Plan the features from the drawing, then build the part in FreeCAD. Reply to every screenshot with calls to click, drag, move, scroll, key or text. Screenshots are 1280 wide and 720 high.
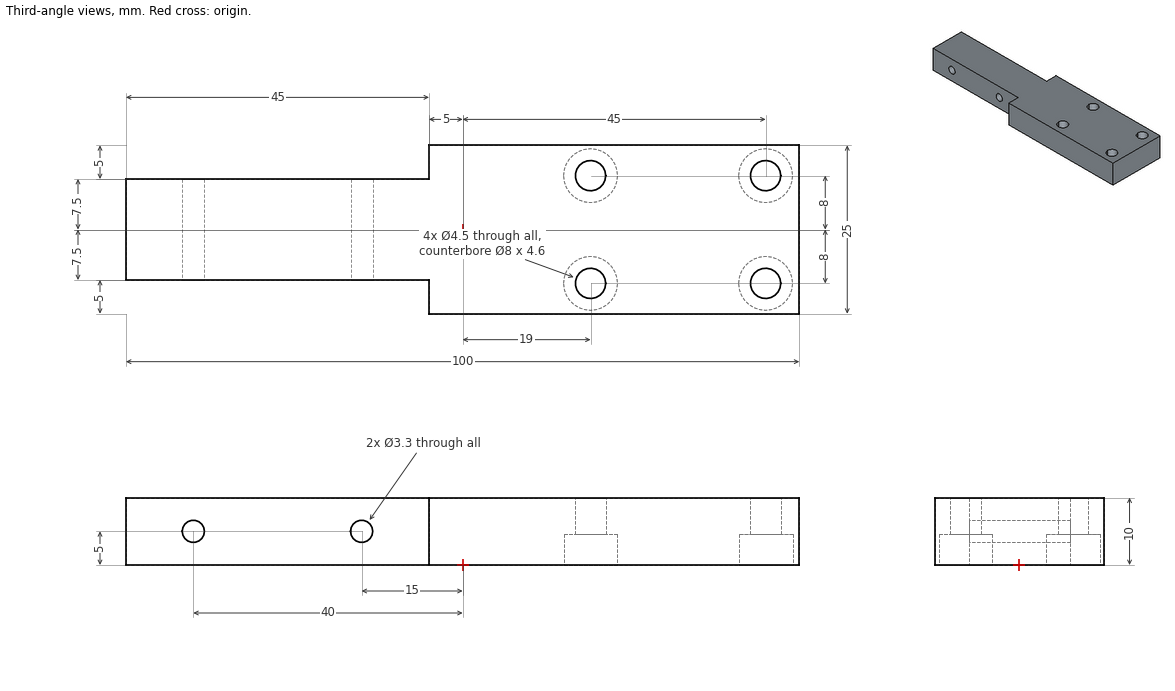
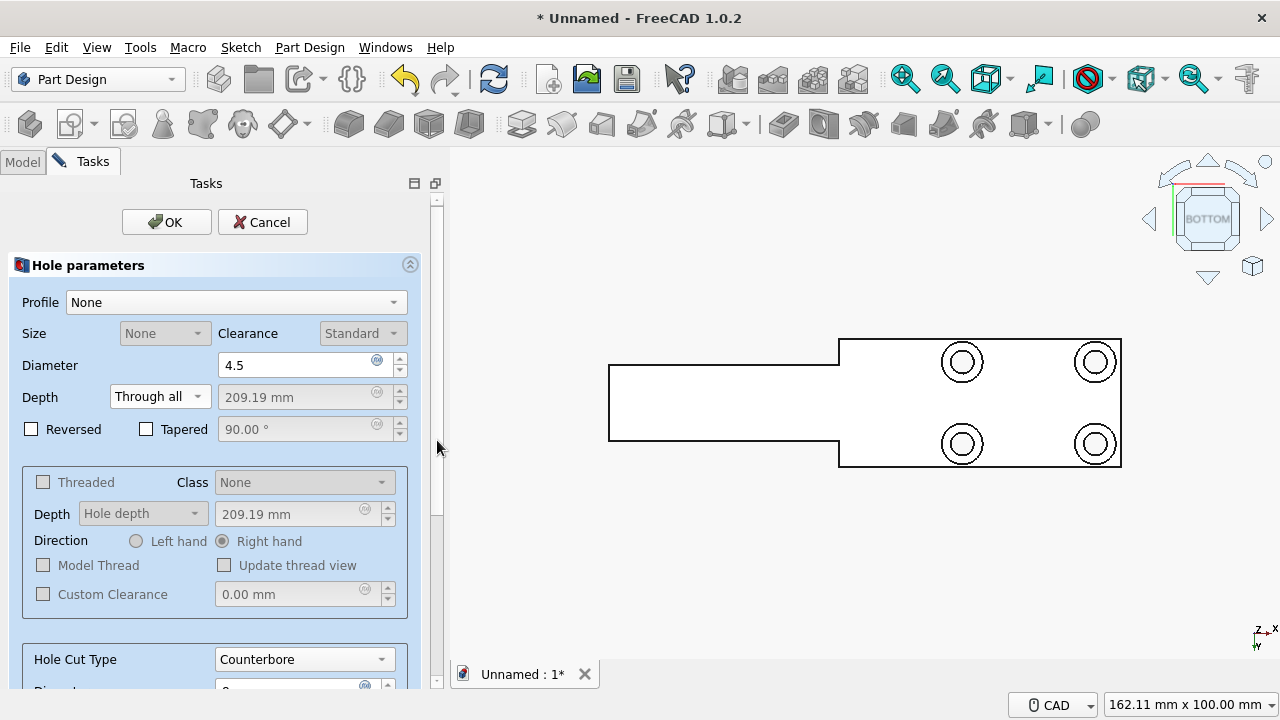
click(167, 222)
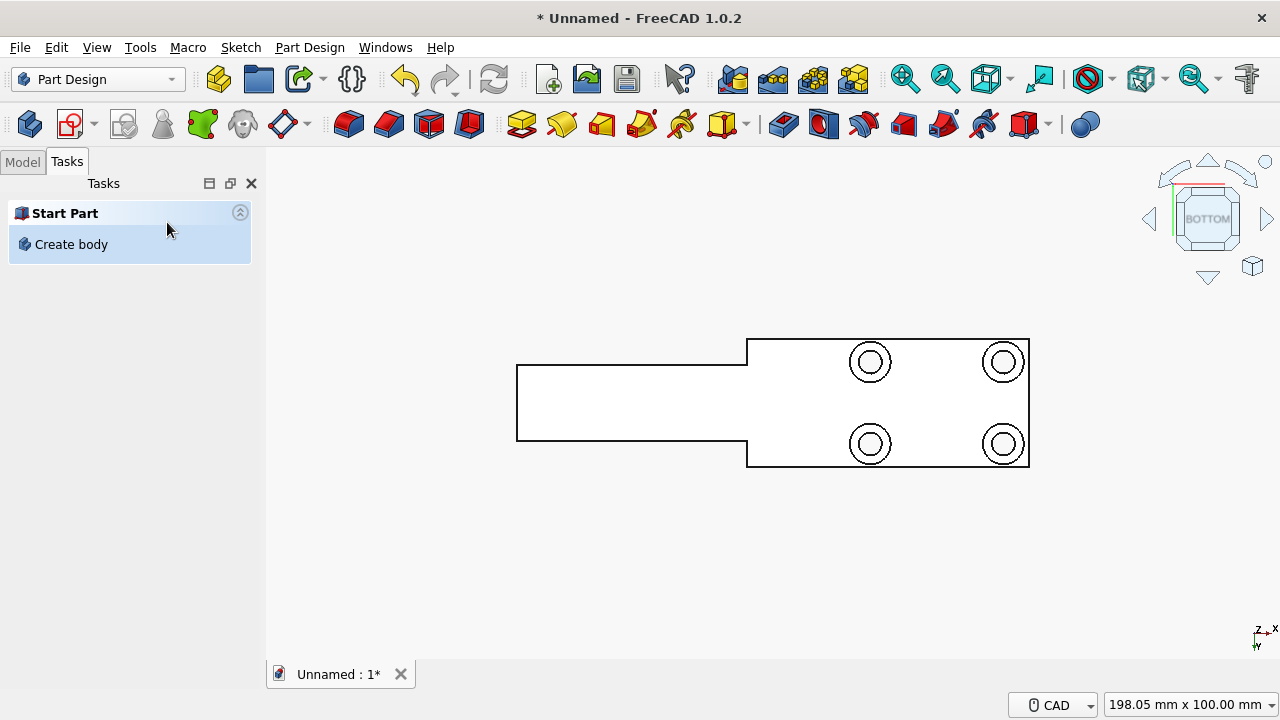
key(4)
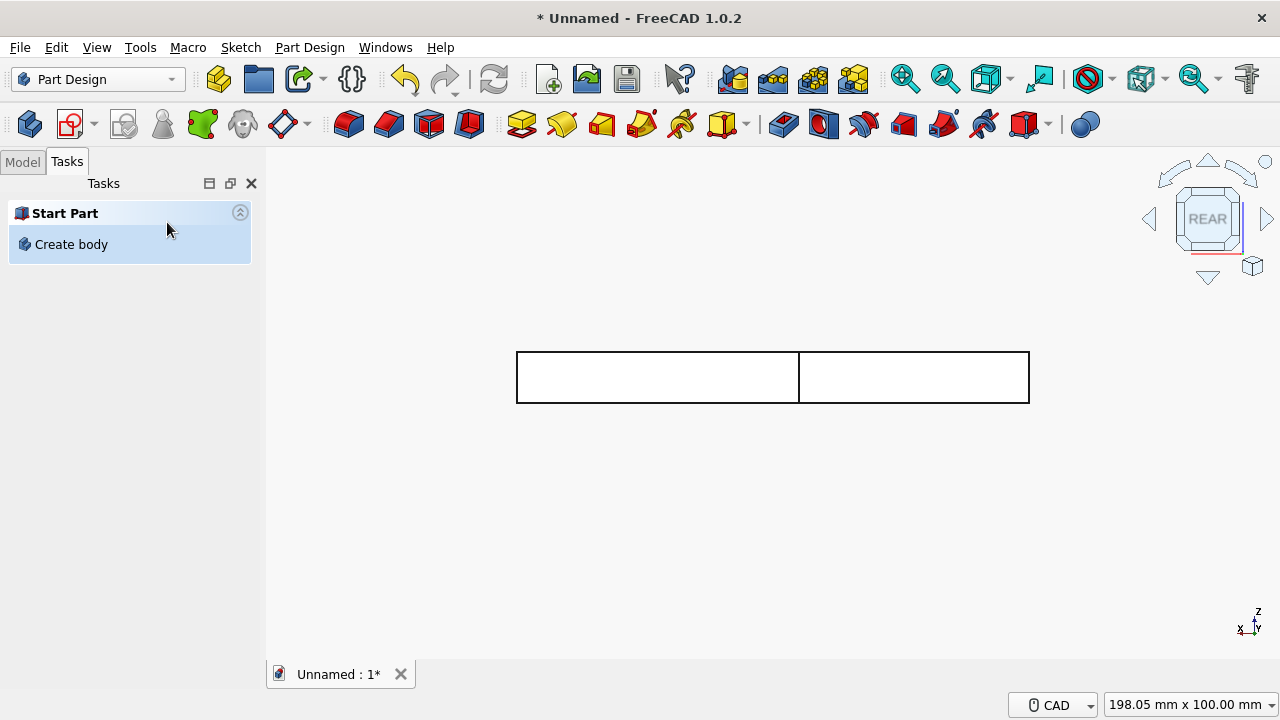
click(848, 376)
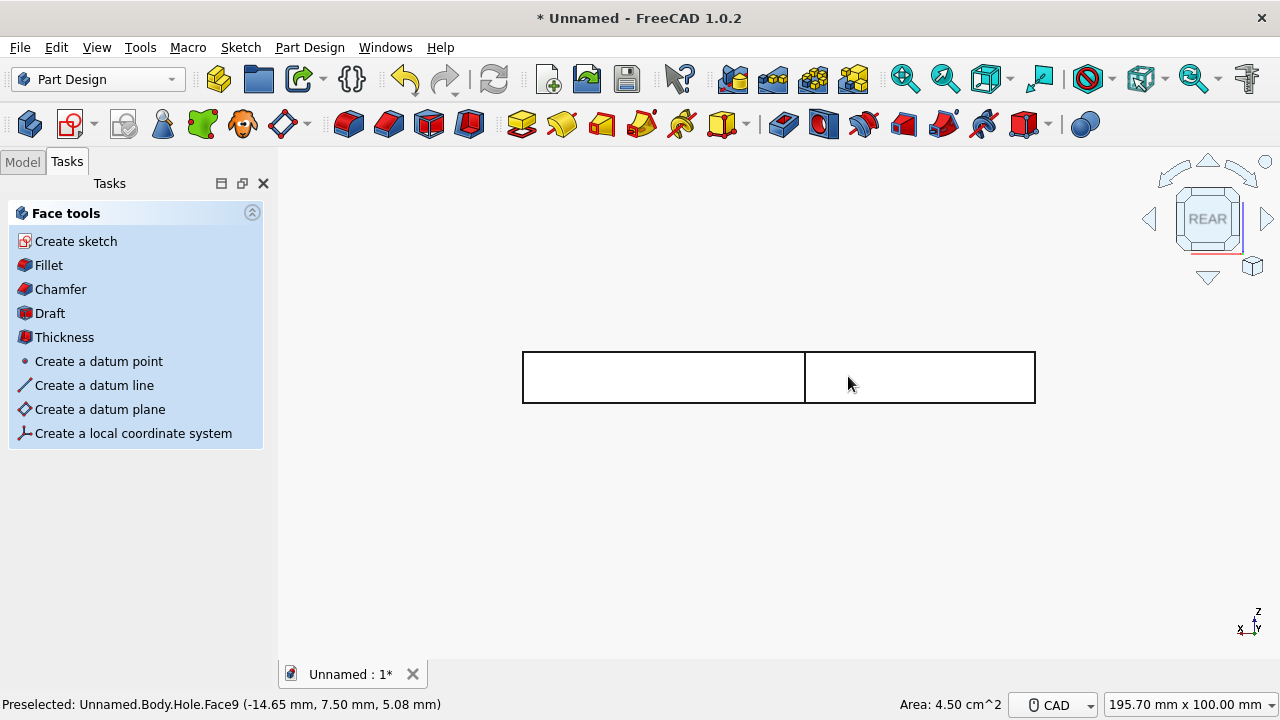
click(70, 124)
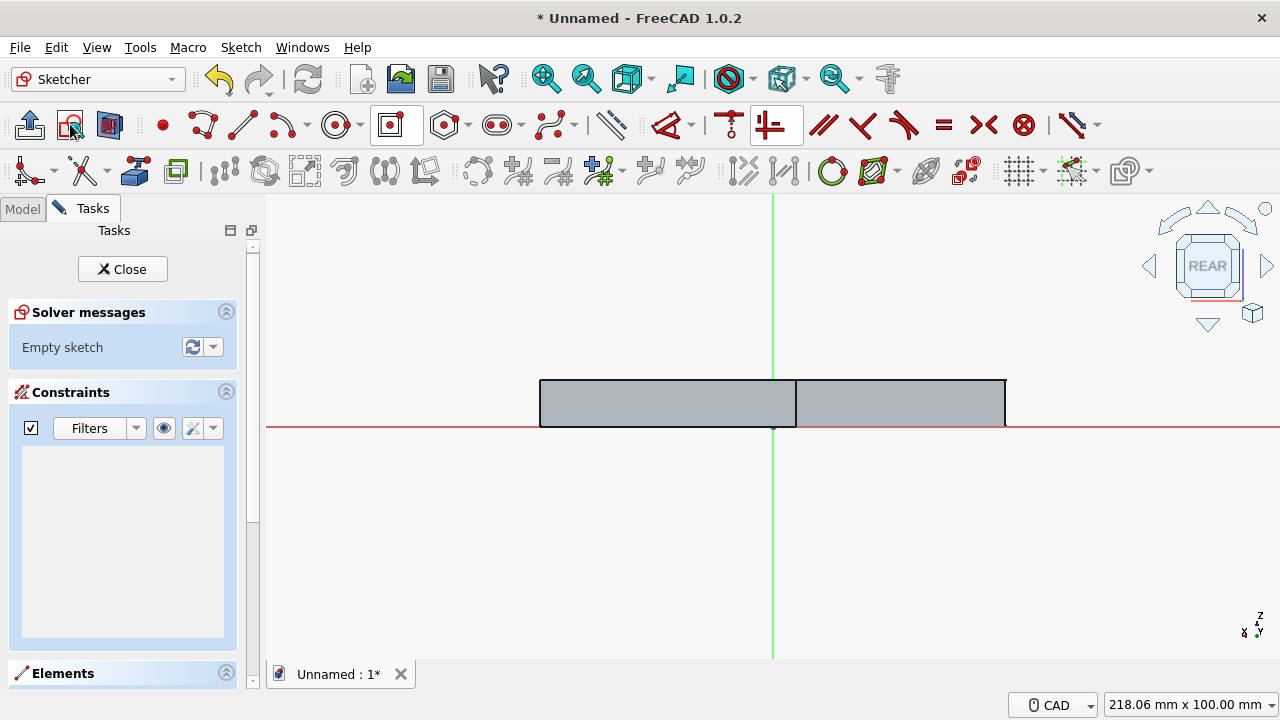
click(110, 126)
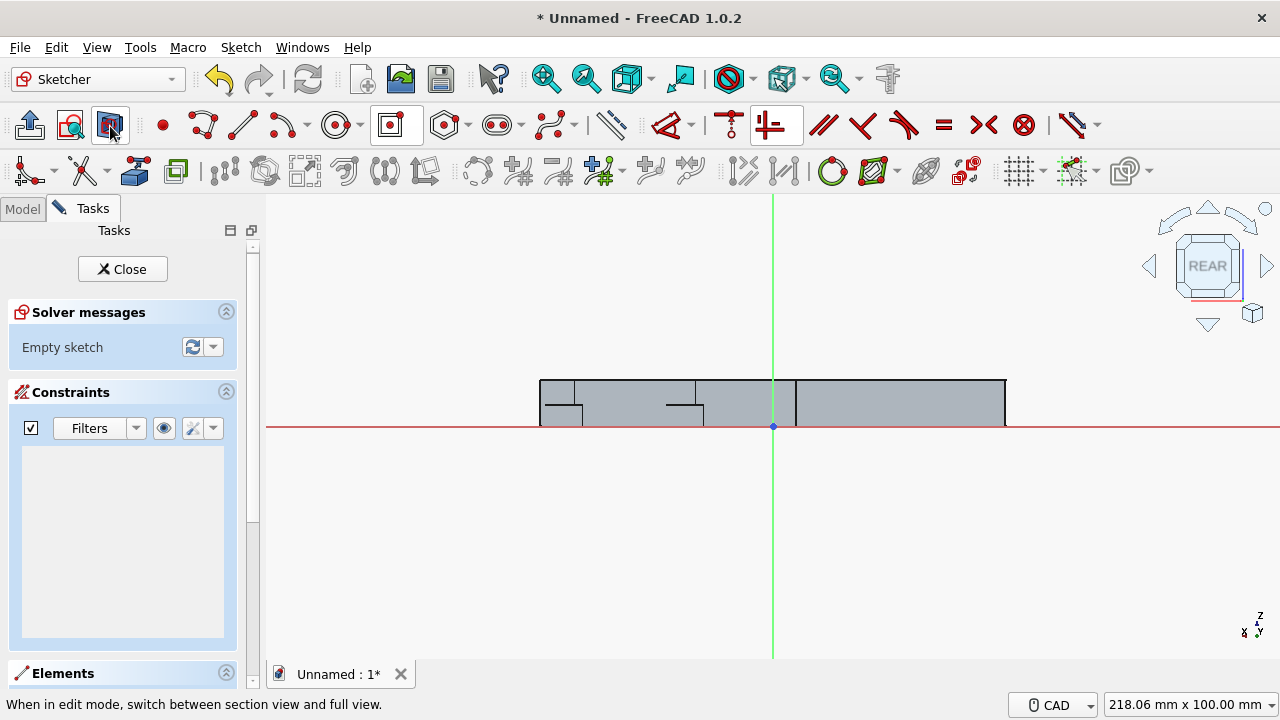
scroll(966, 402, up, 5)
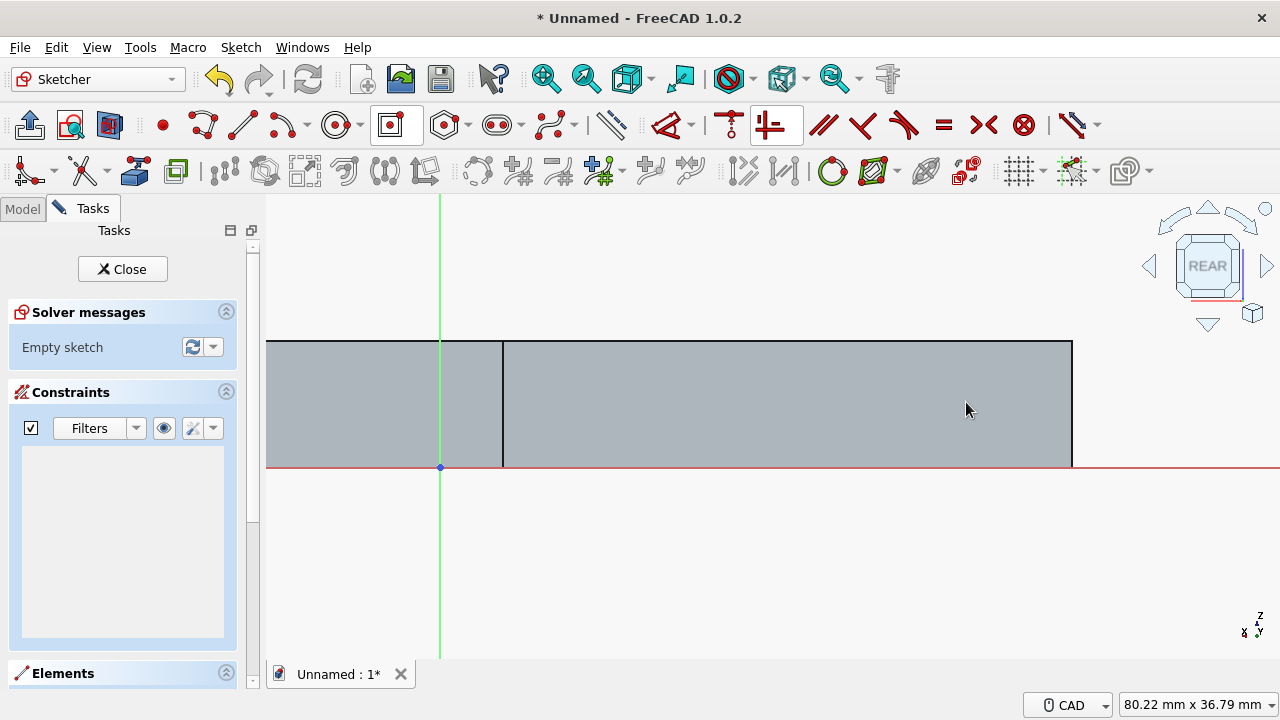
click(336, 126)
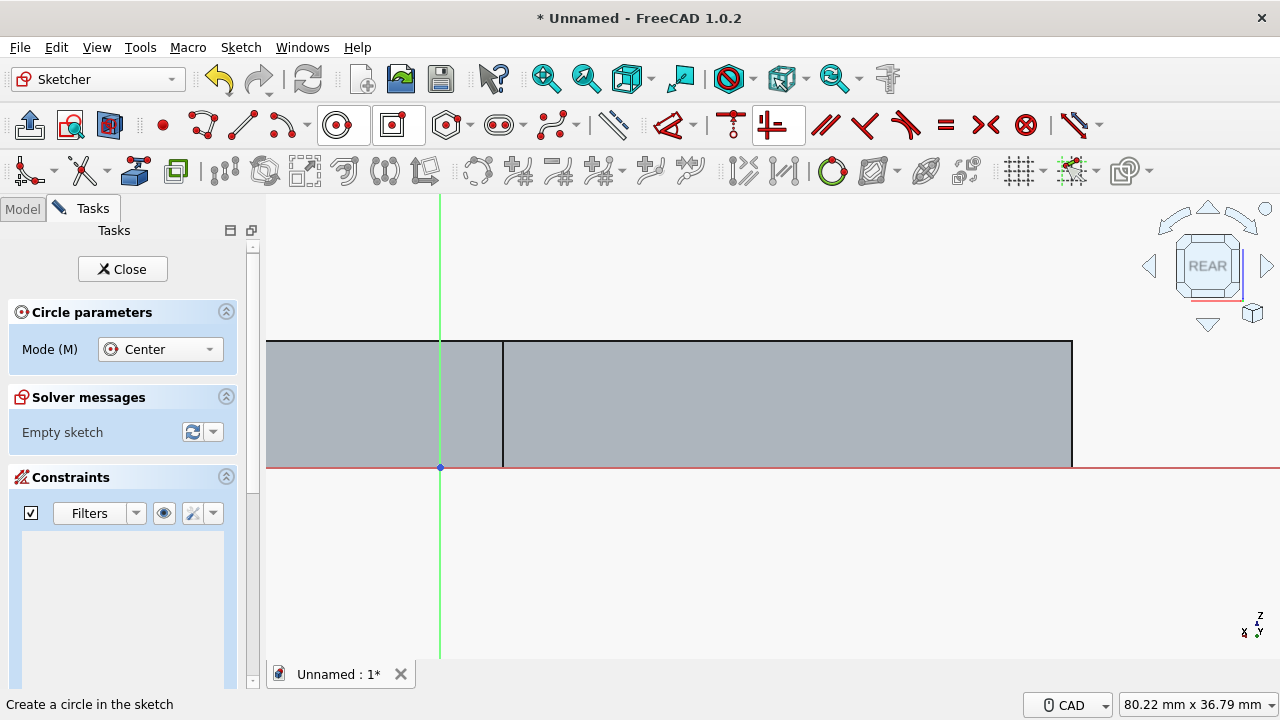
click(630, 405)
click(645, 390)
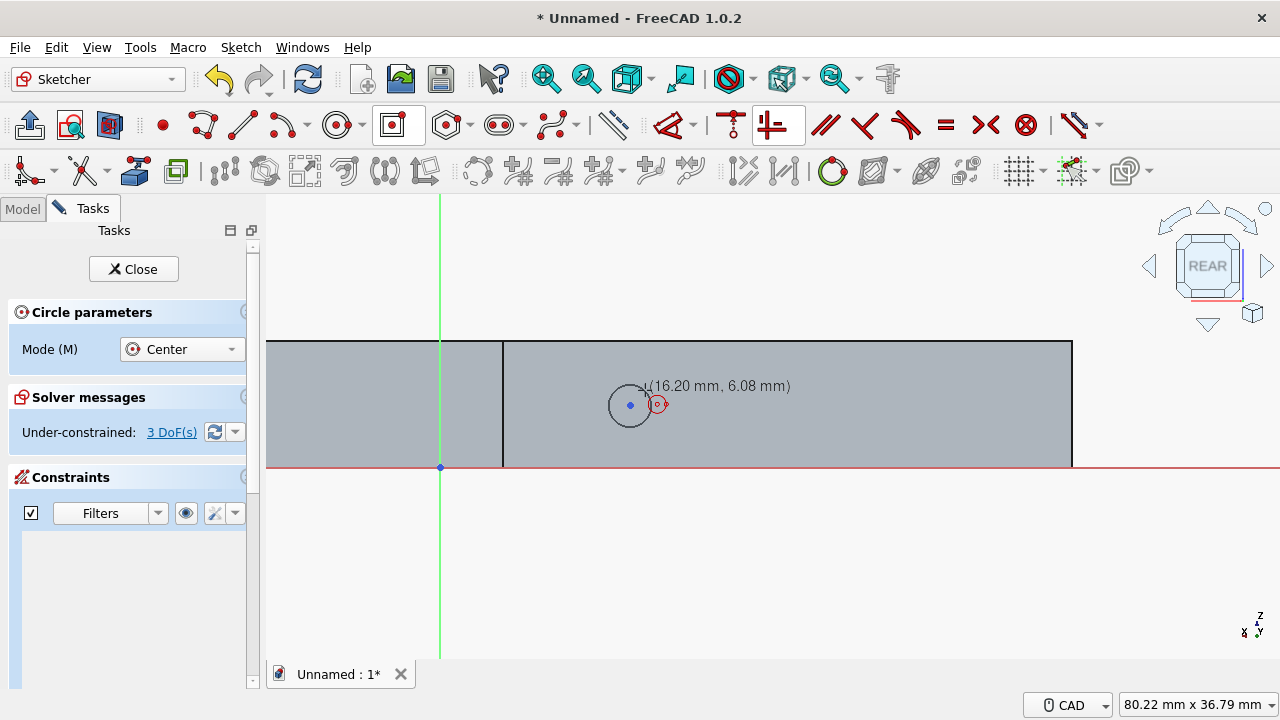
click(946, 405)
click(961, 390)
key(Escape)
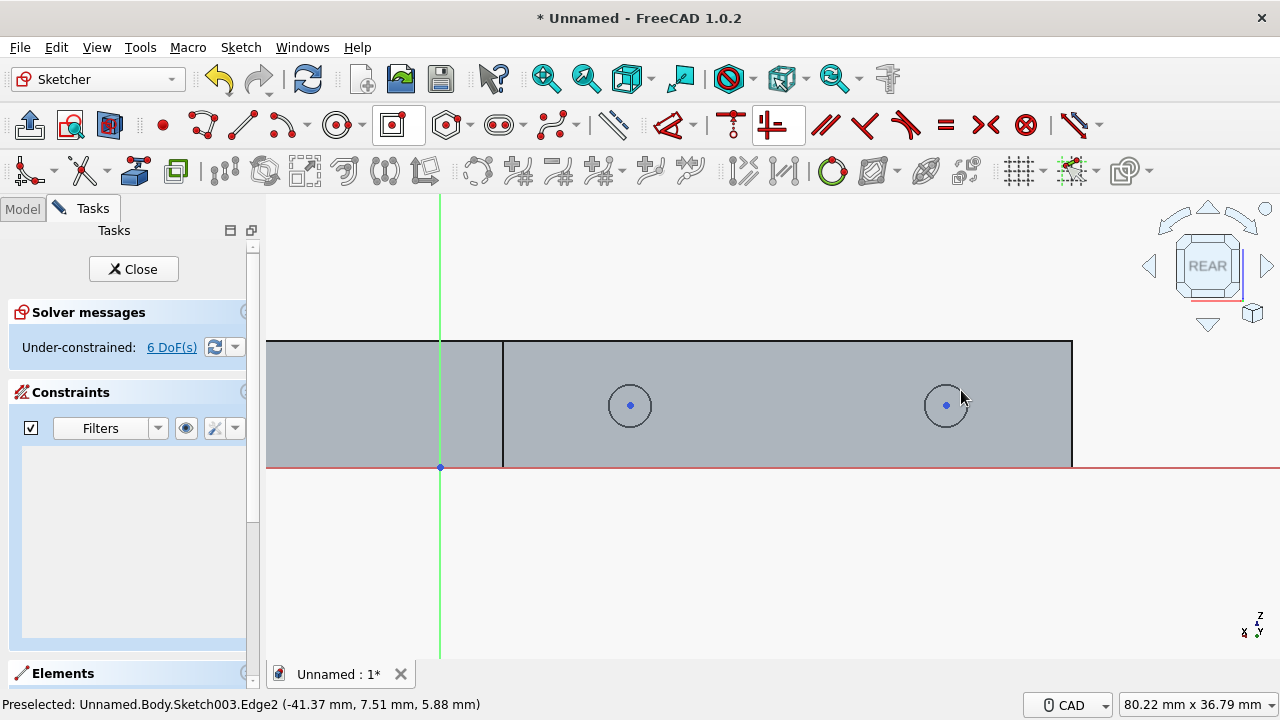
click(645, 391)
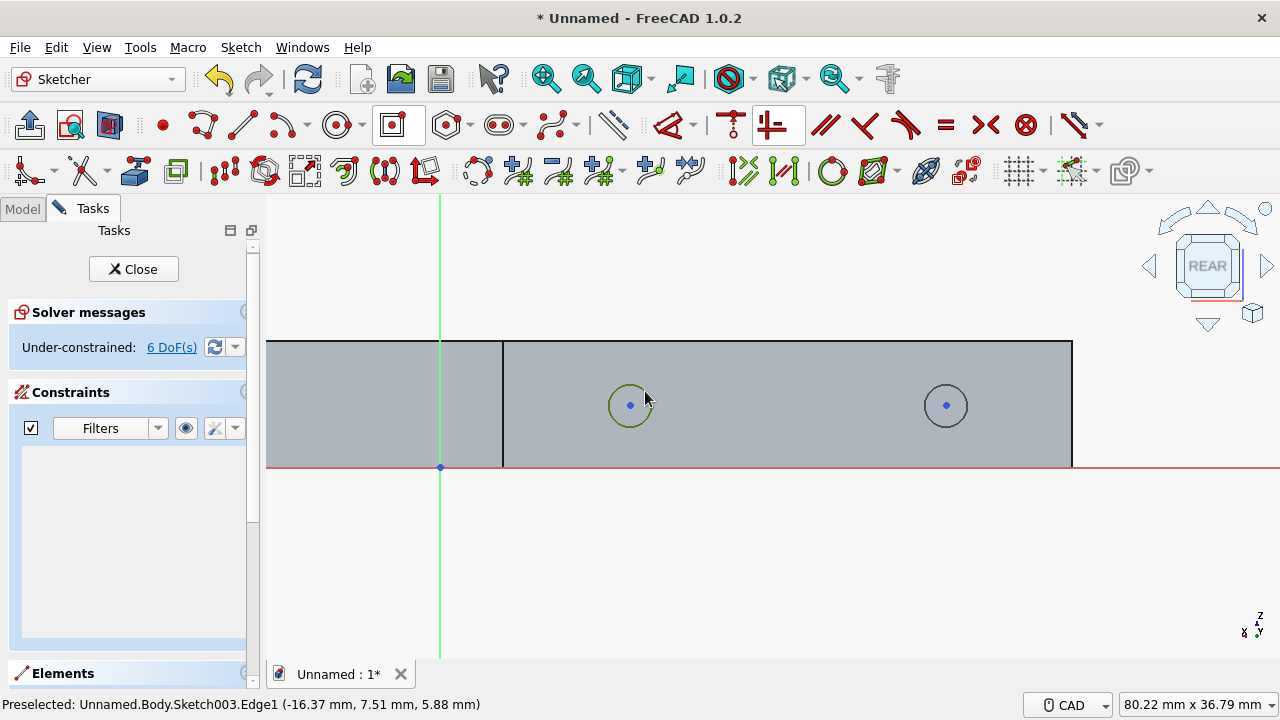
click(961, 391)